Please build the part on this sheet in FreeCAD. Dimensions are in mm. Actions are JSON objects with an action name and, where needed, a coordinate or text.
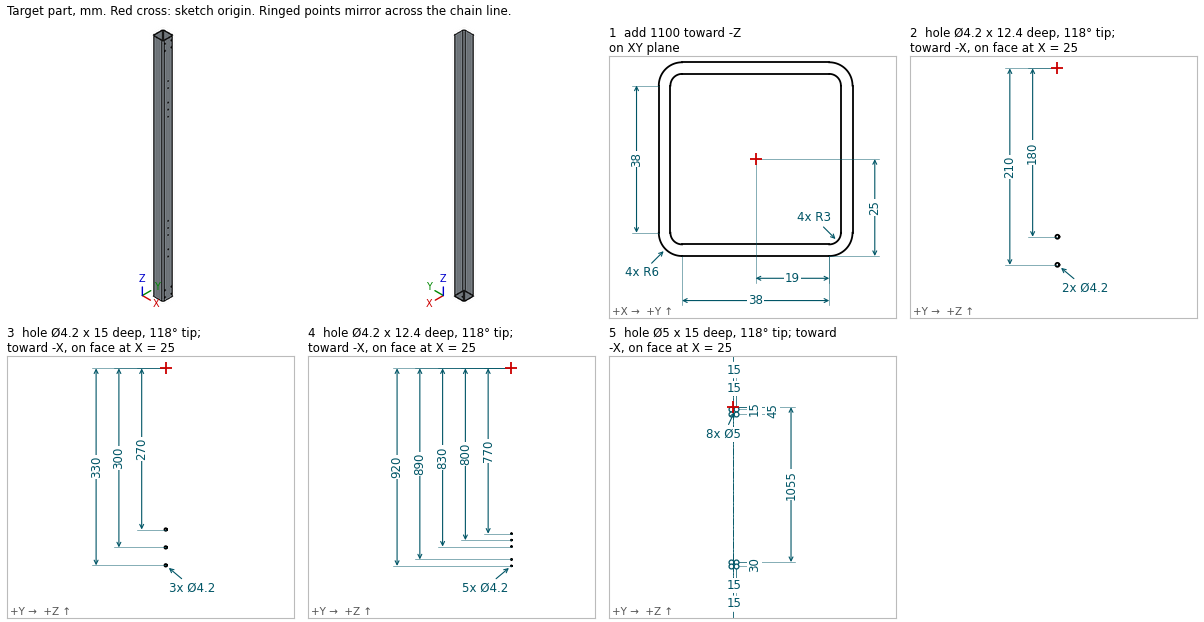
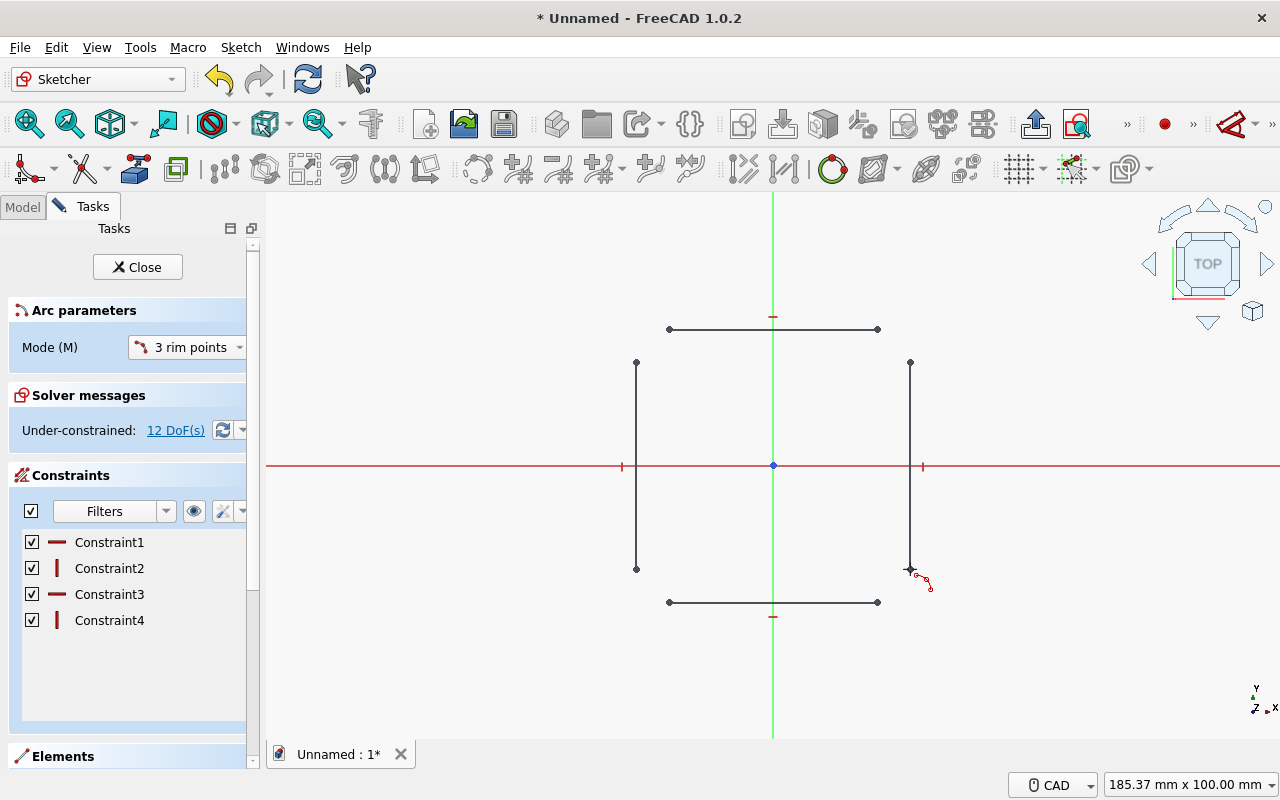
{"action": "left_click", "coordinate": [669, 603]}
{"action": "left_click", "coordinate": [636, 570]}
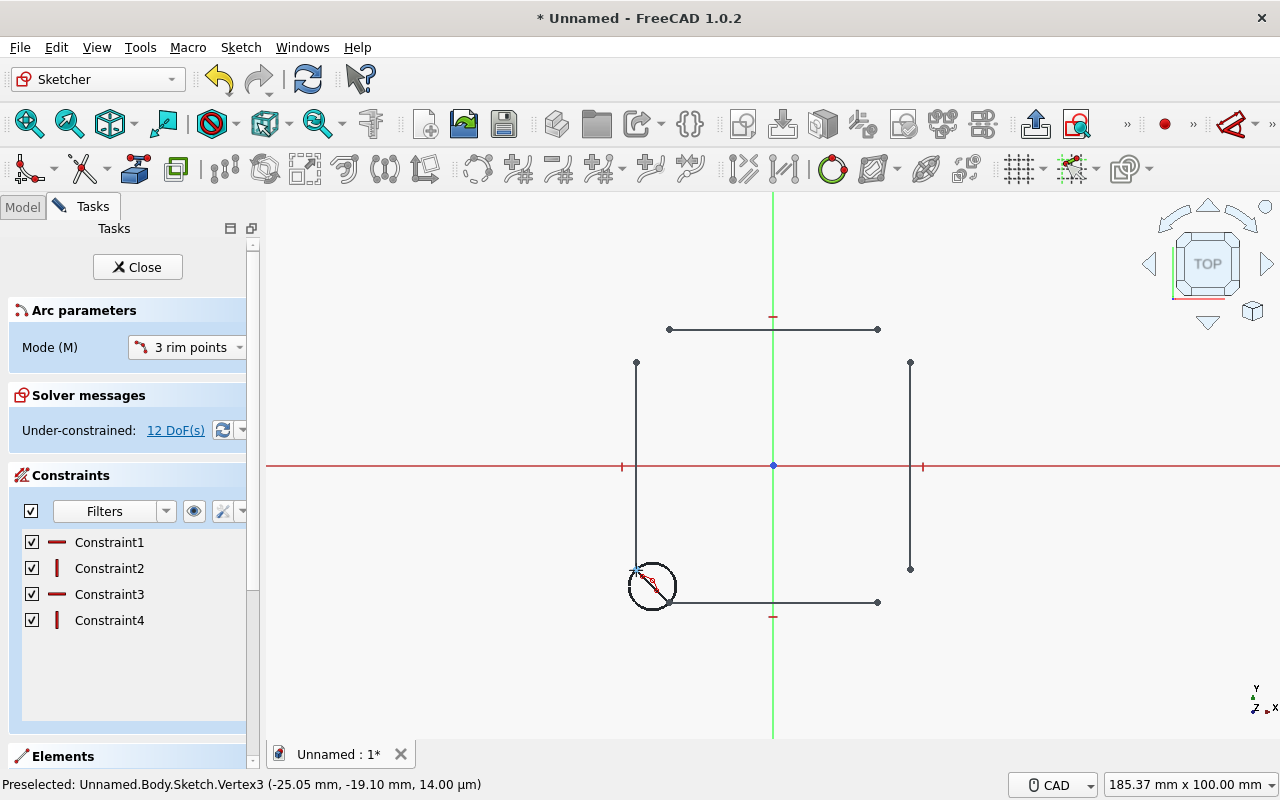
{"action": "scroll", "coordinate": [646, 593], "scroll_direction": "up", "scroll_amount": 3}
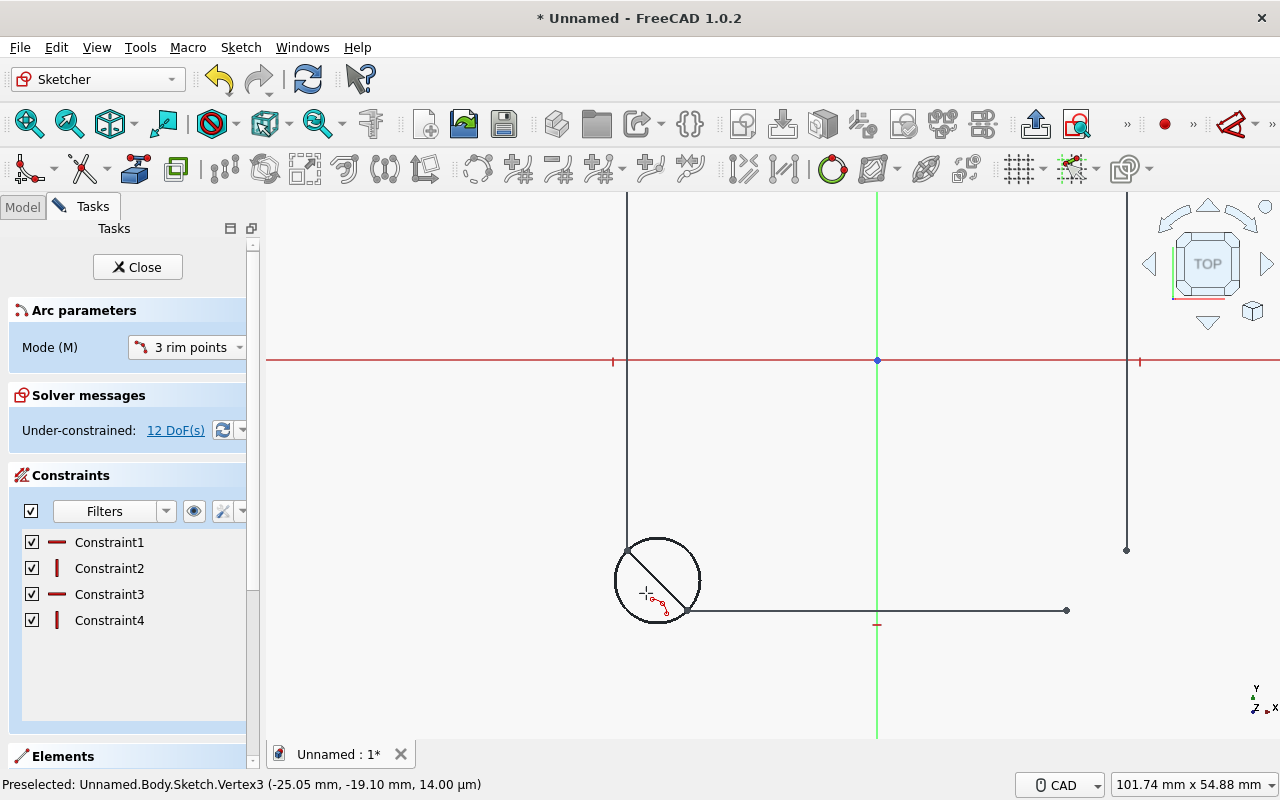
{"action": "left_click", "coordinate": [645, 592]}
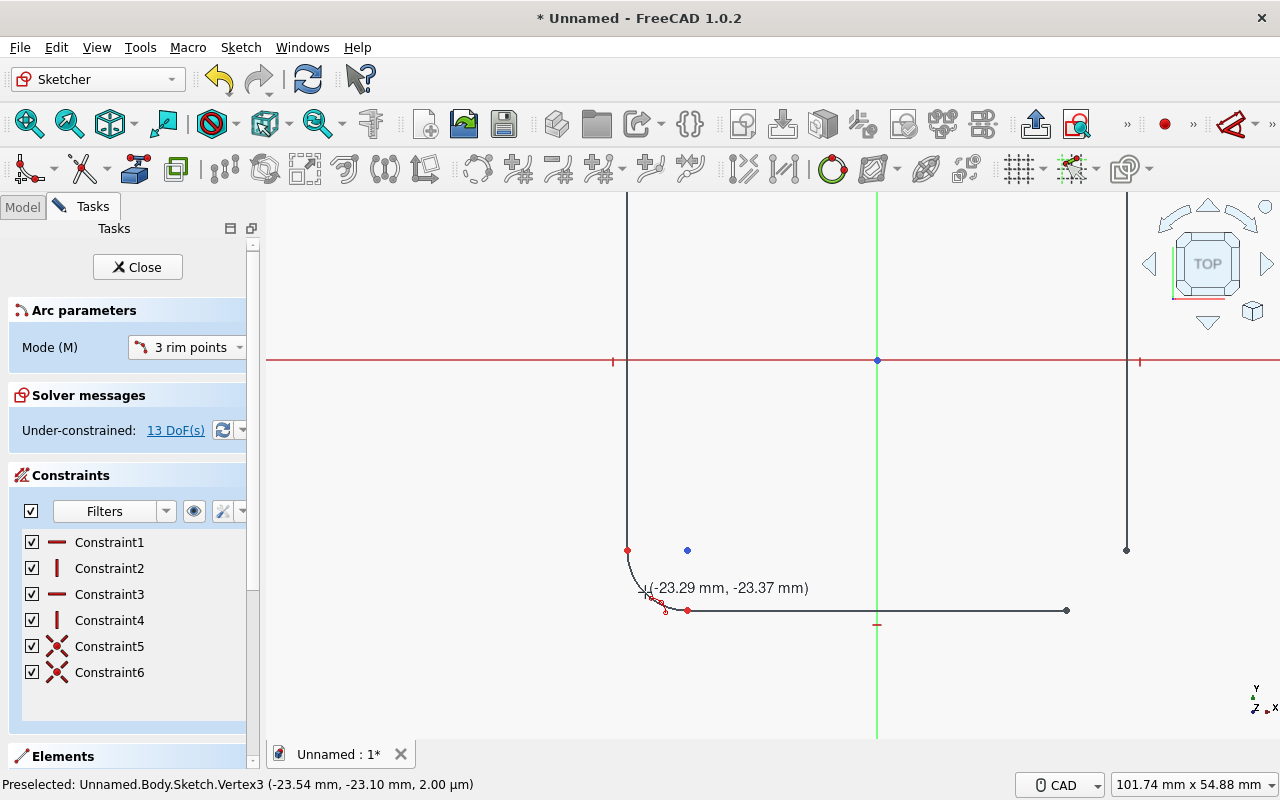
{"action": "scroll", "coordinate": [354, 680], "scroll_direction": "down", "scroll_amount": 2}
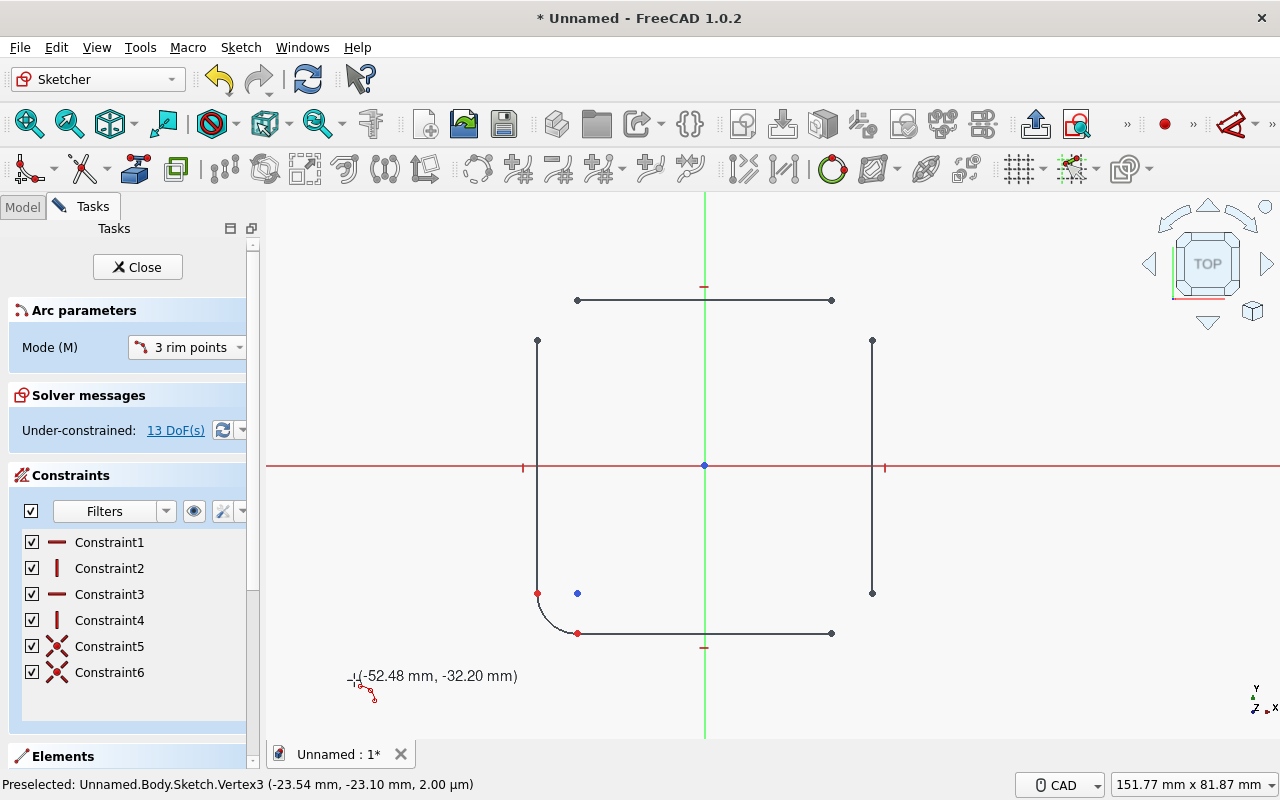
{"action": "left_click", "coordinate": [537, 341]}
{"action": "left_click", "coordinate": [578, 300]}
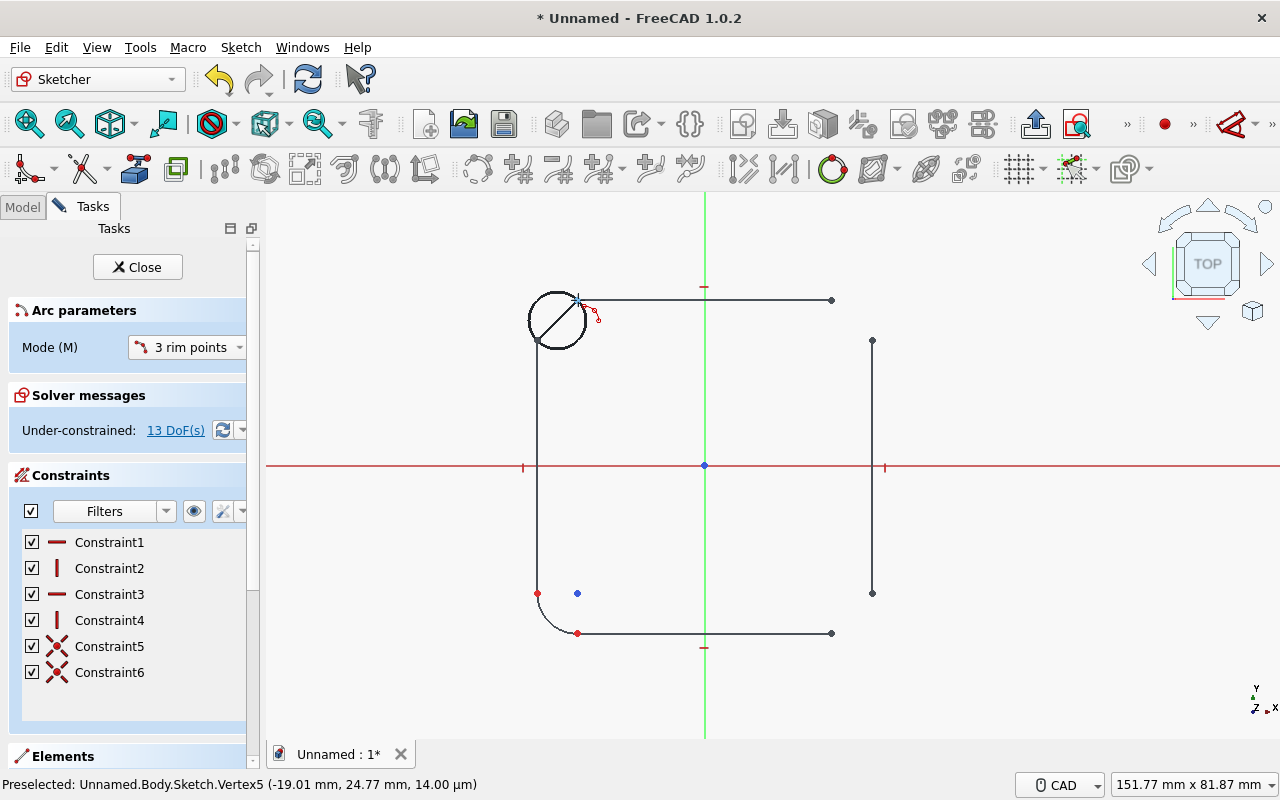
{"action": "scroll", "coordinate": [549, 311], "scroll_direction": "up", "scroll_amount": 2}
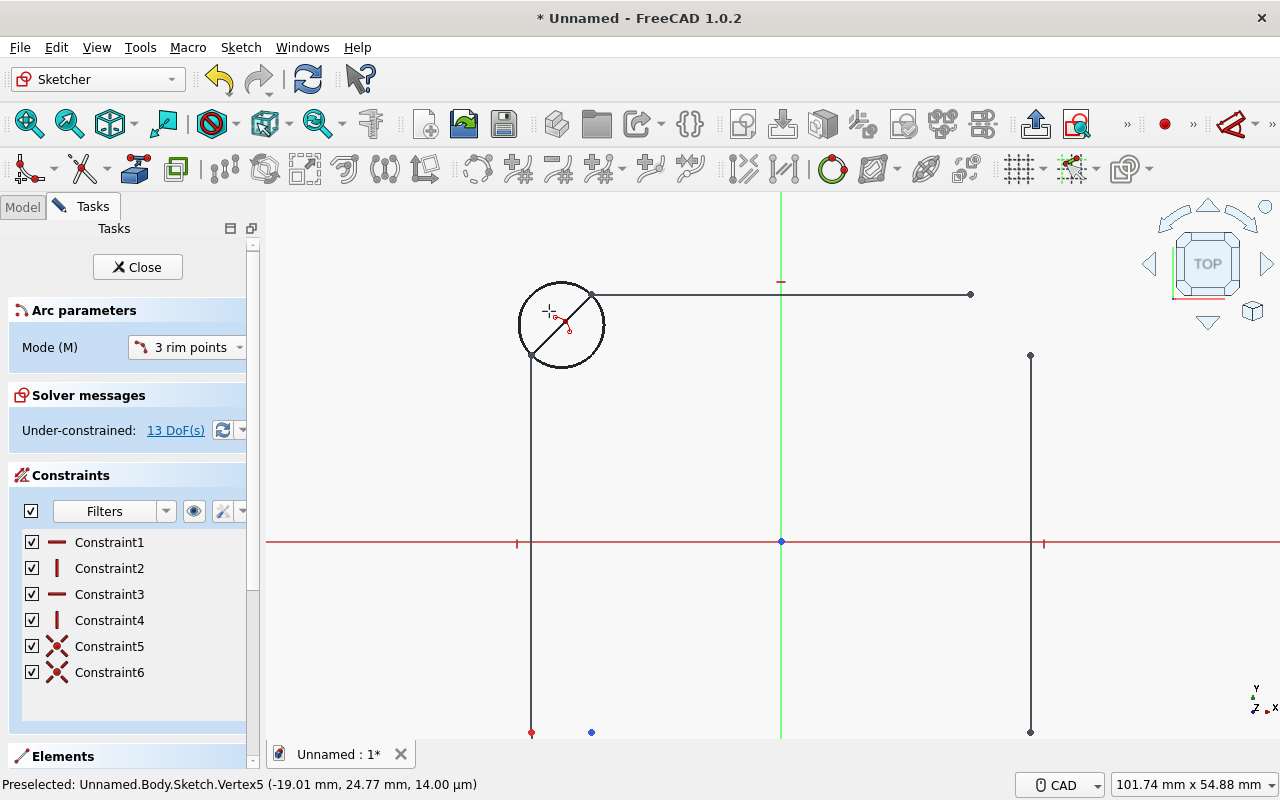
{"action": "left_click", "coordinate": [549, 310]}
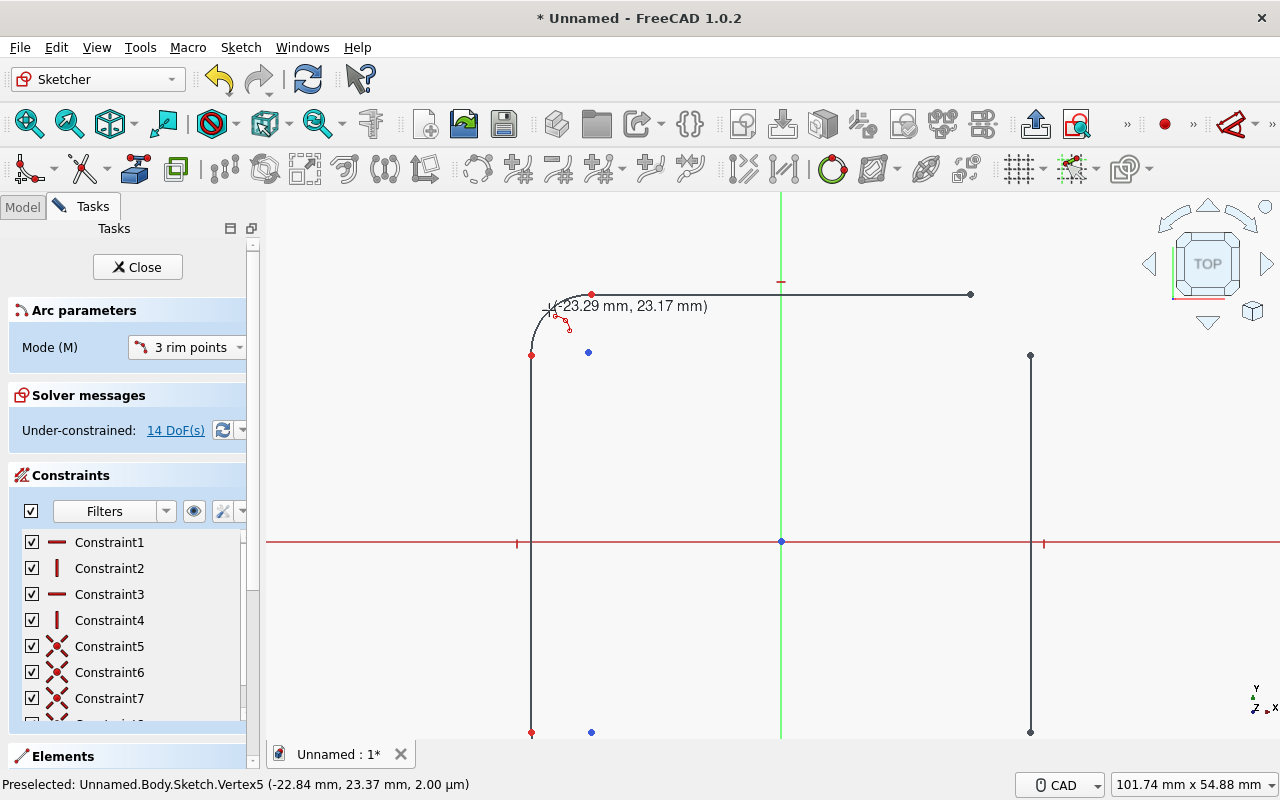
{"action": "left_click", "coordinate": [971, 295]}
{"action": "left_click", "coordinate": [1031, 355]}
{"action": "left_click", "coordinate": [1013, 310]}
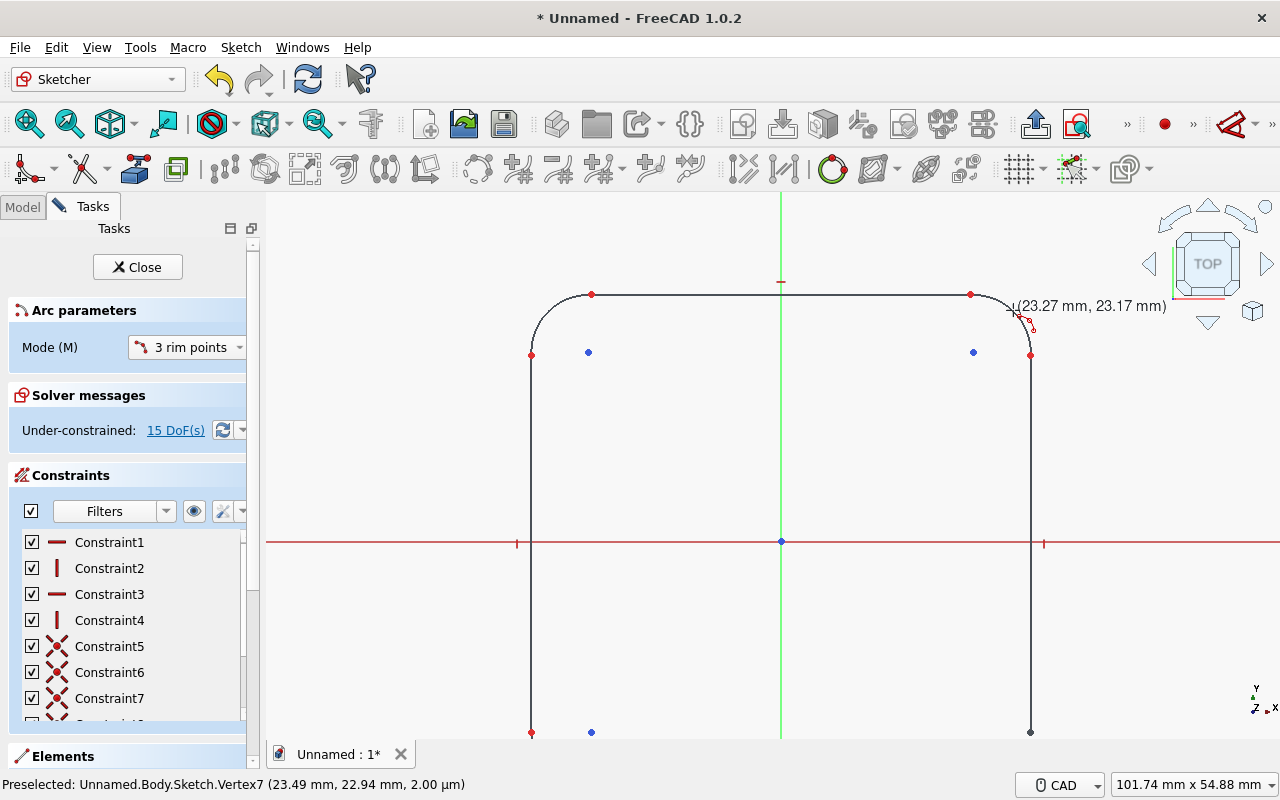
{"action": "scroll", "coordinate": [549, 310], "scroll_direction": "down", "scroll_amount": 2}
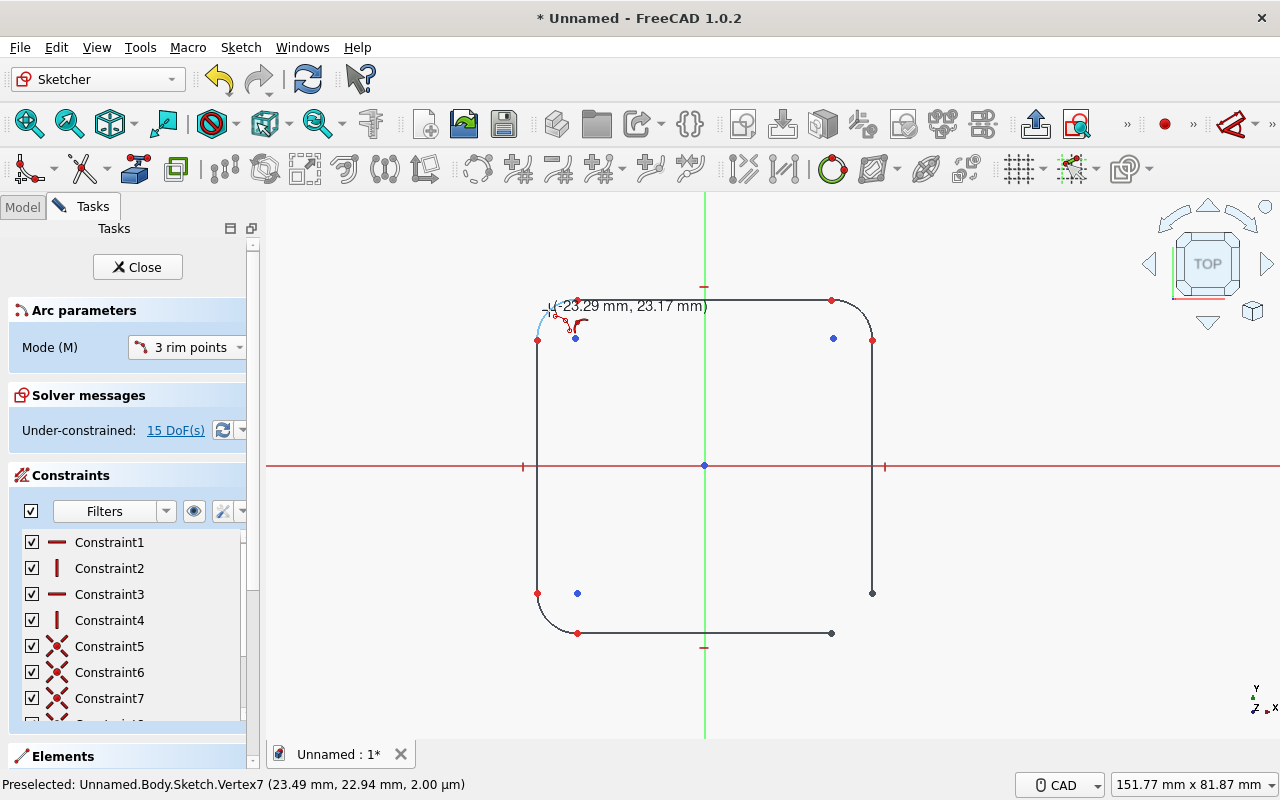
{"action": "left_click", "coordinate": [872, 593]}
{"action": "left_click", "coordinate": [832, 633]}